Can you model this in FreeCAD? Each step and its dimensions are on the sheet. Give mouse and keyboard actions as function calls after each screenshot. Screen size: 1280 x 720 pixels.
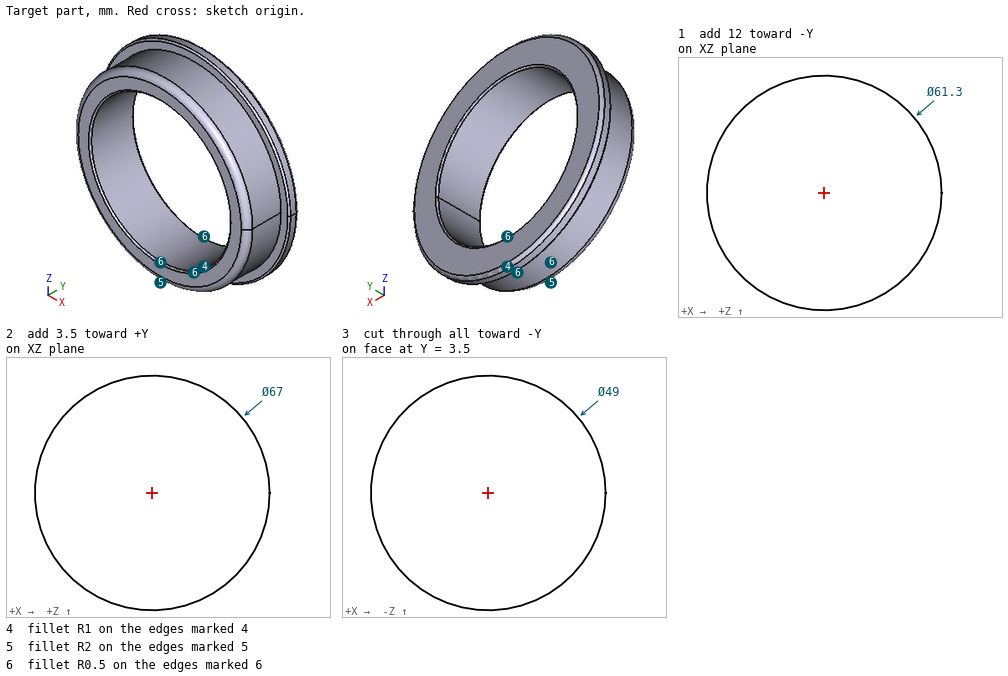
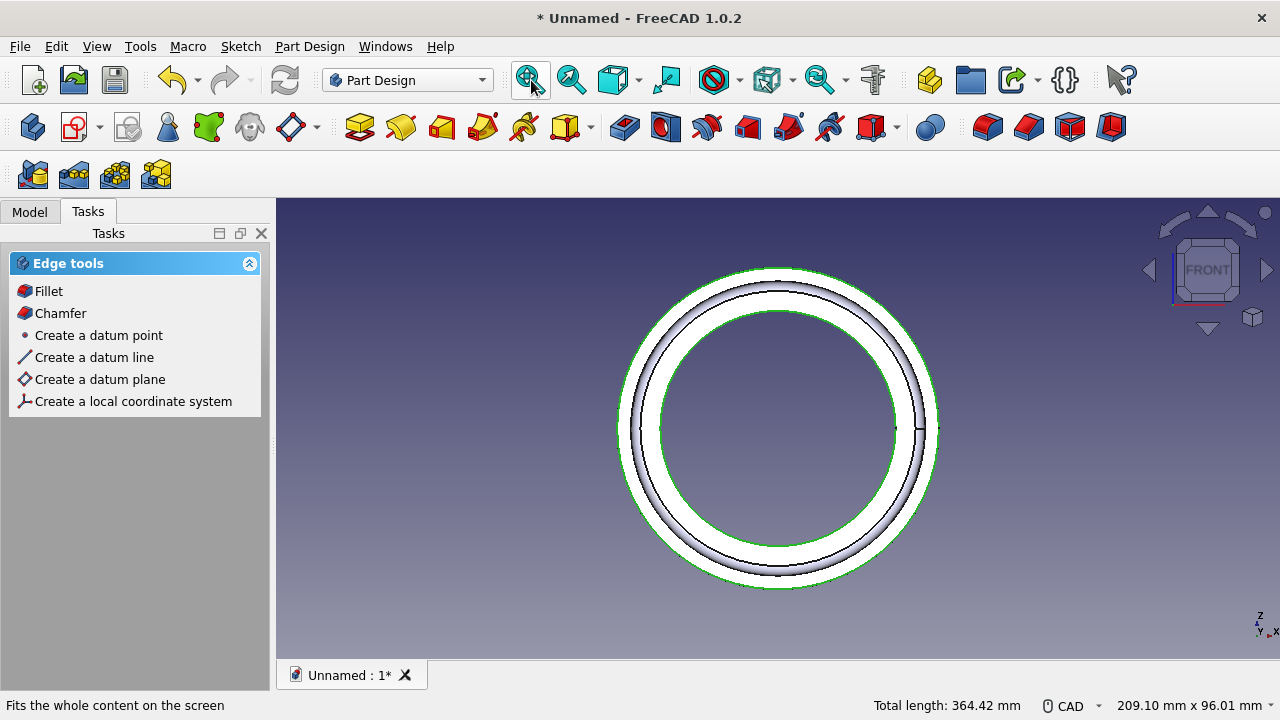
key(3)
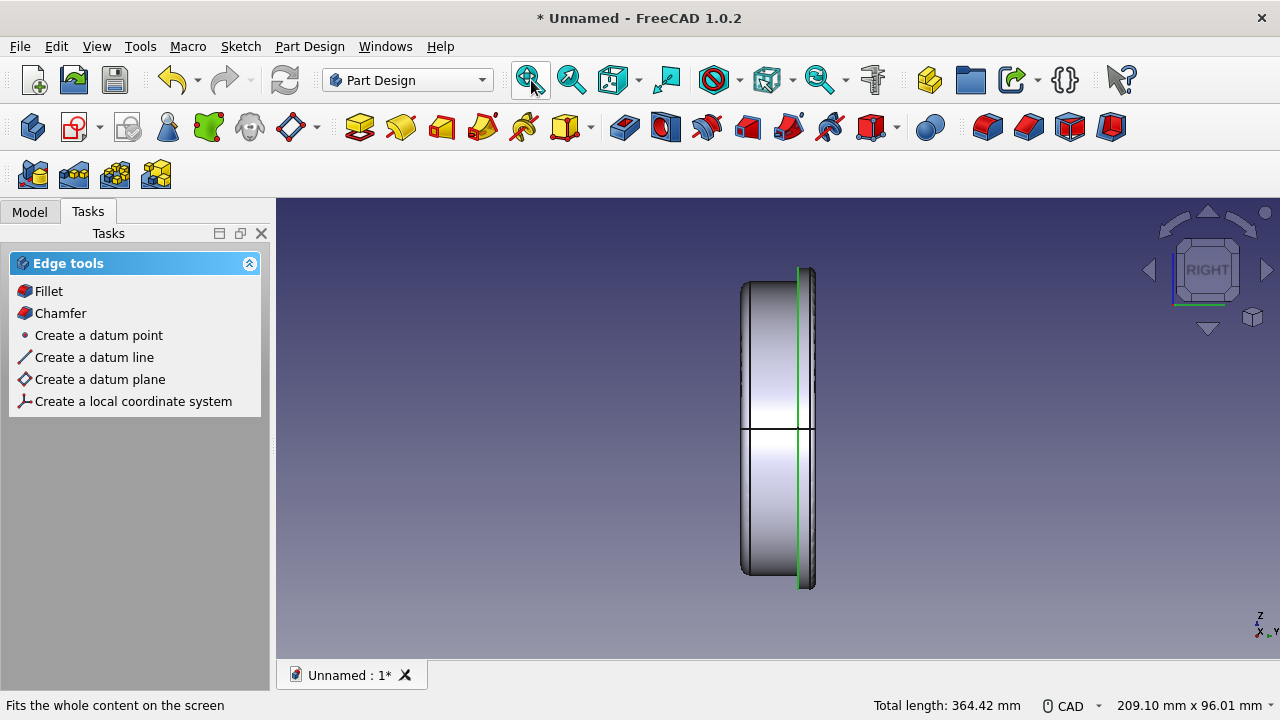
key(5)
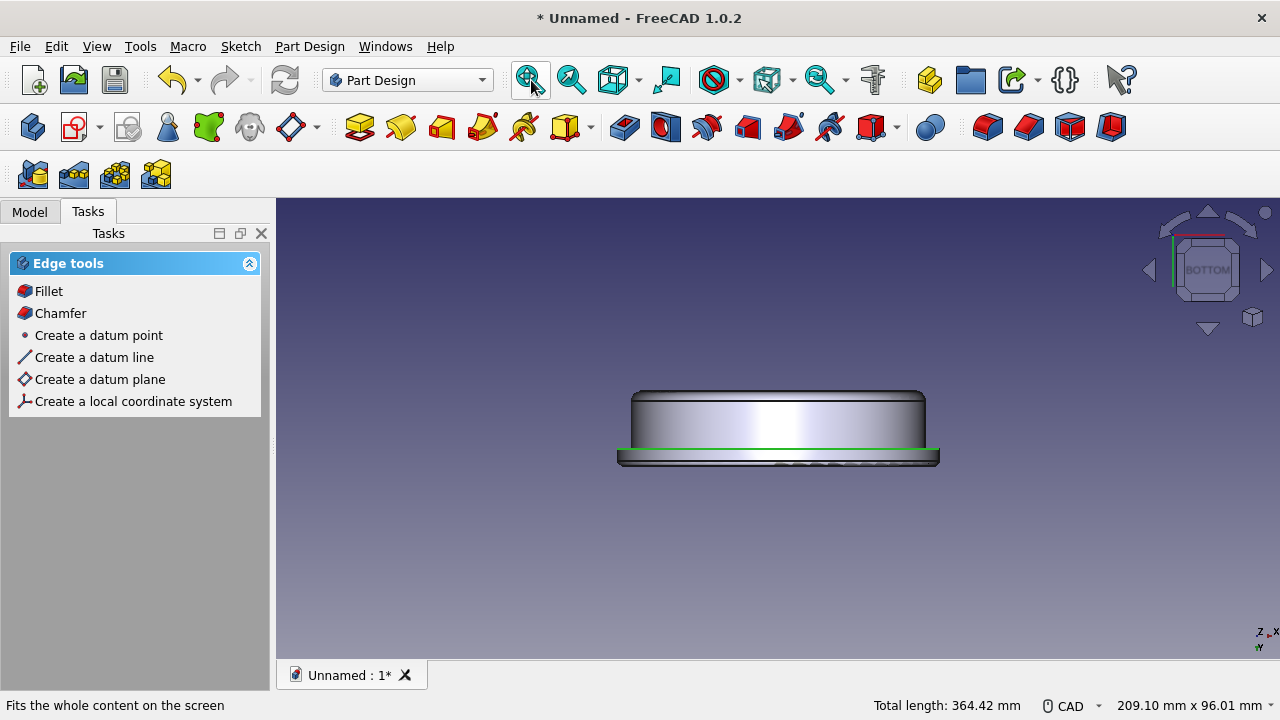
click(531, 80)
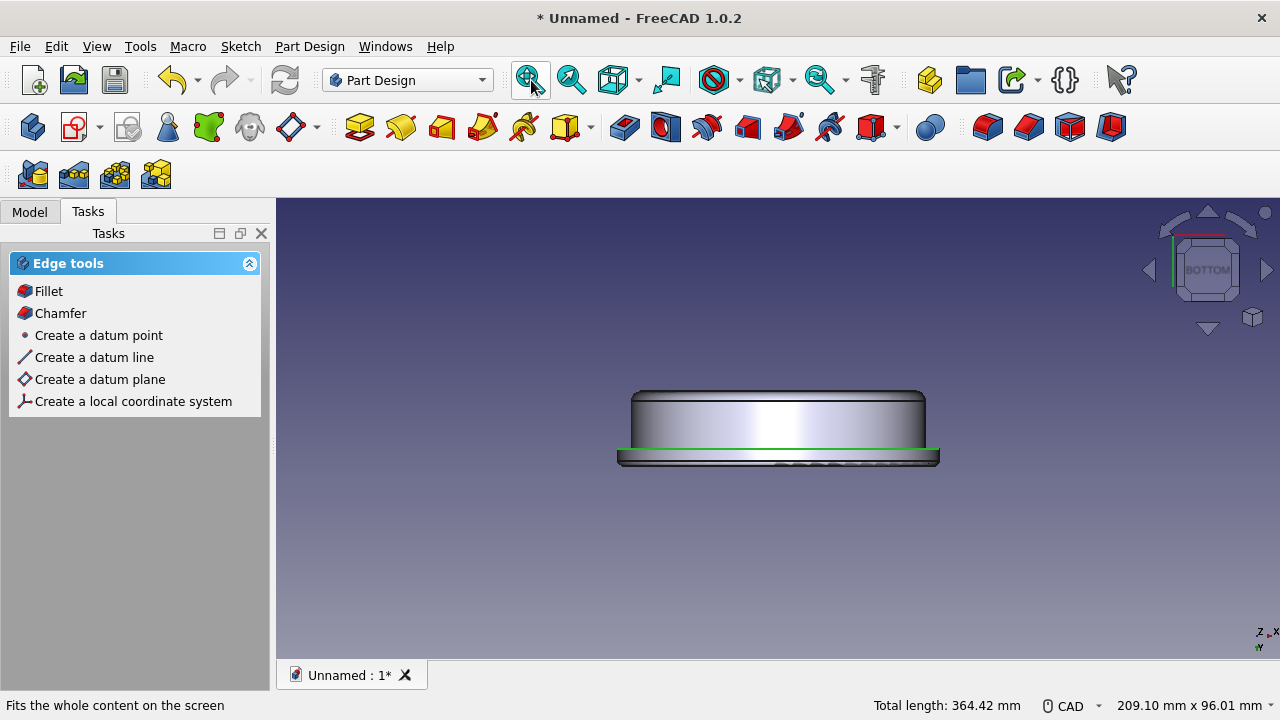
key(4)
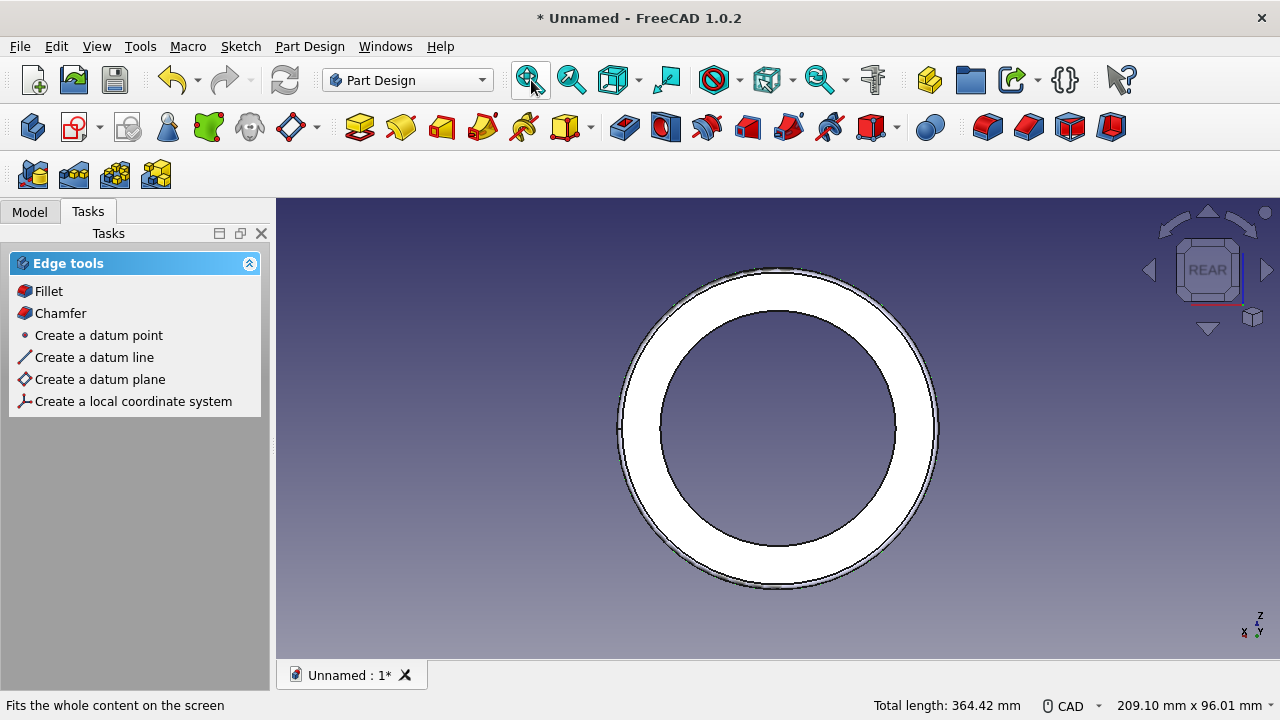
click(873, 358, ctrl)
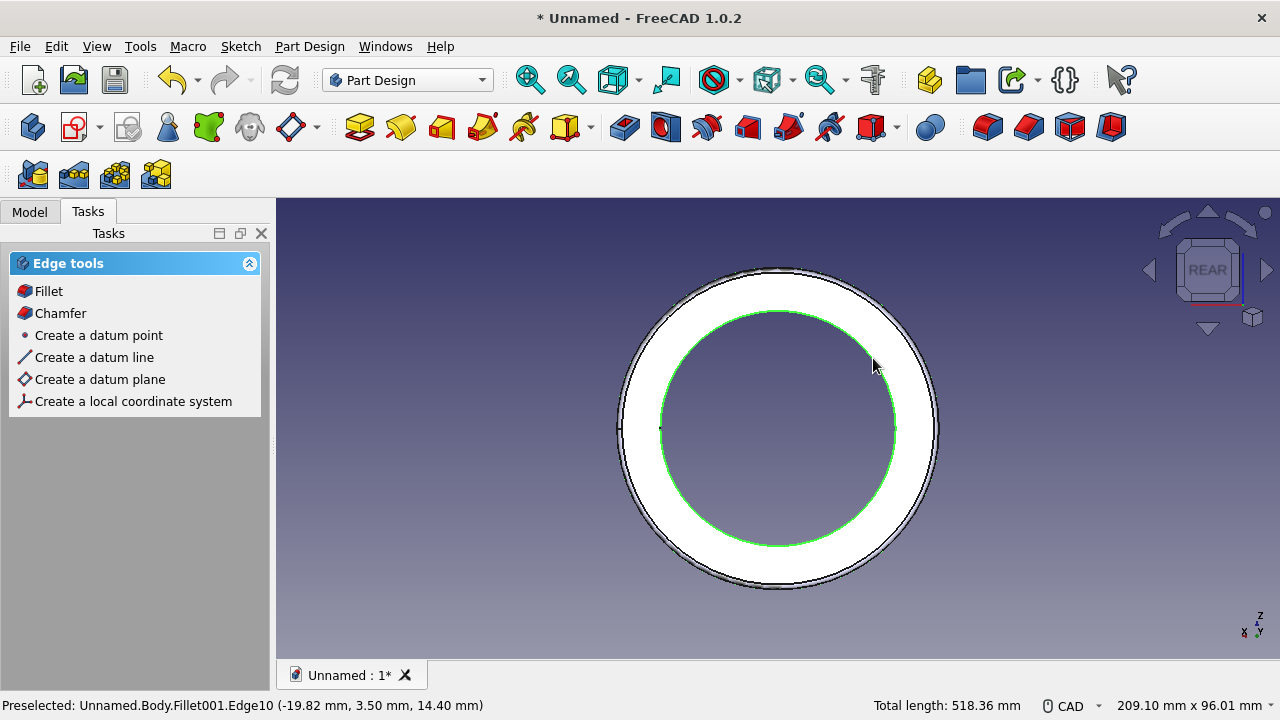
click(988, 128)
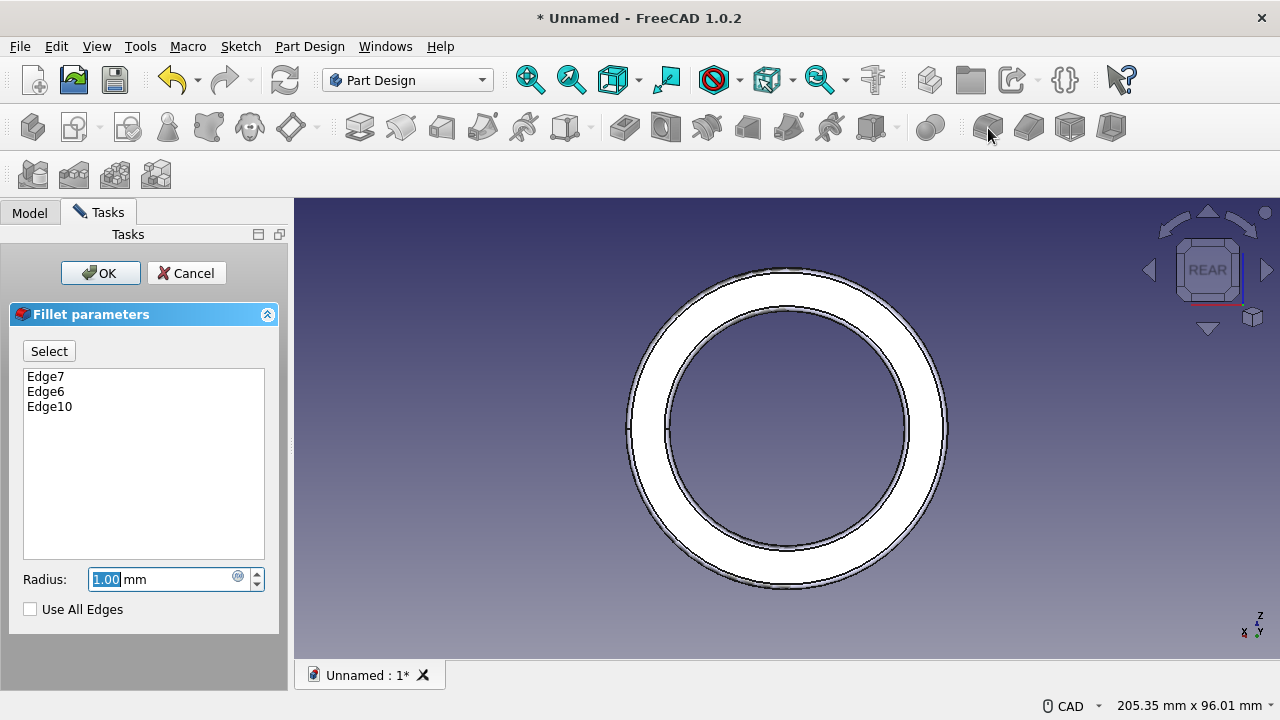
text(0.5)
key(Tab)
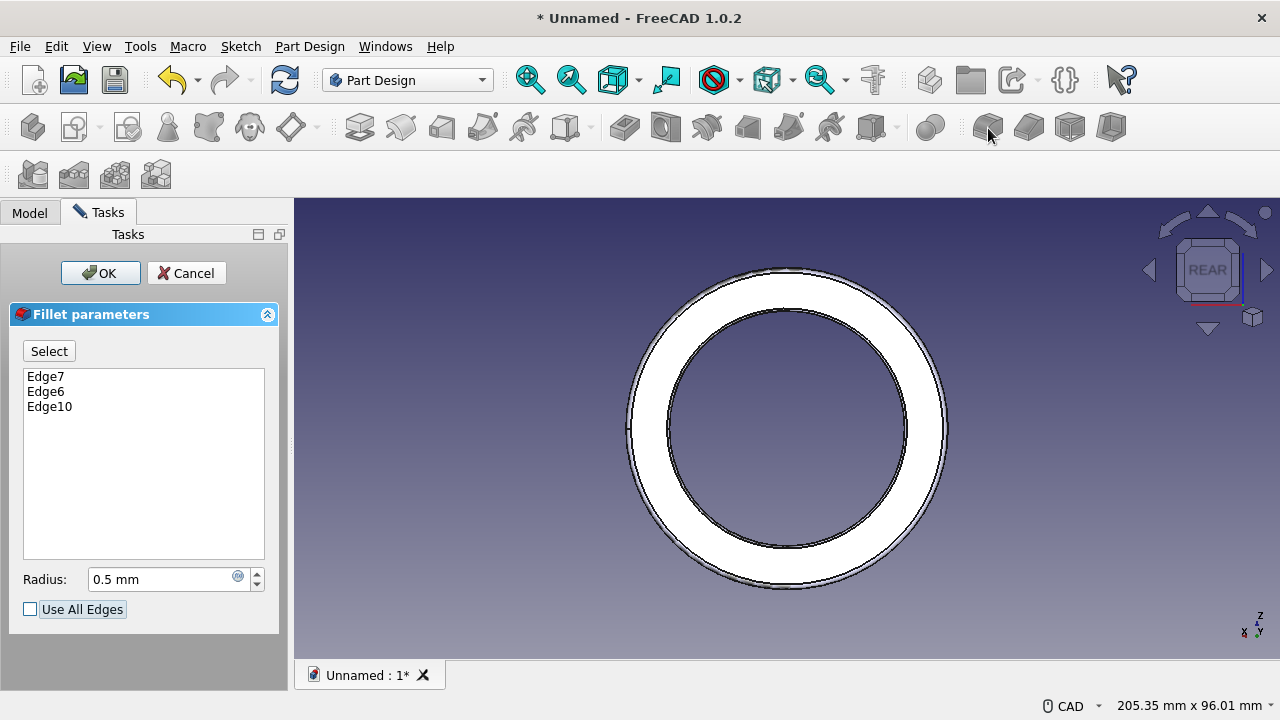
click(101, 273)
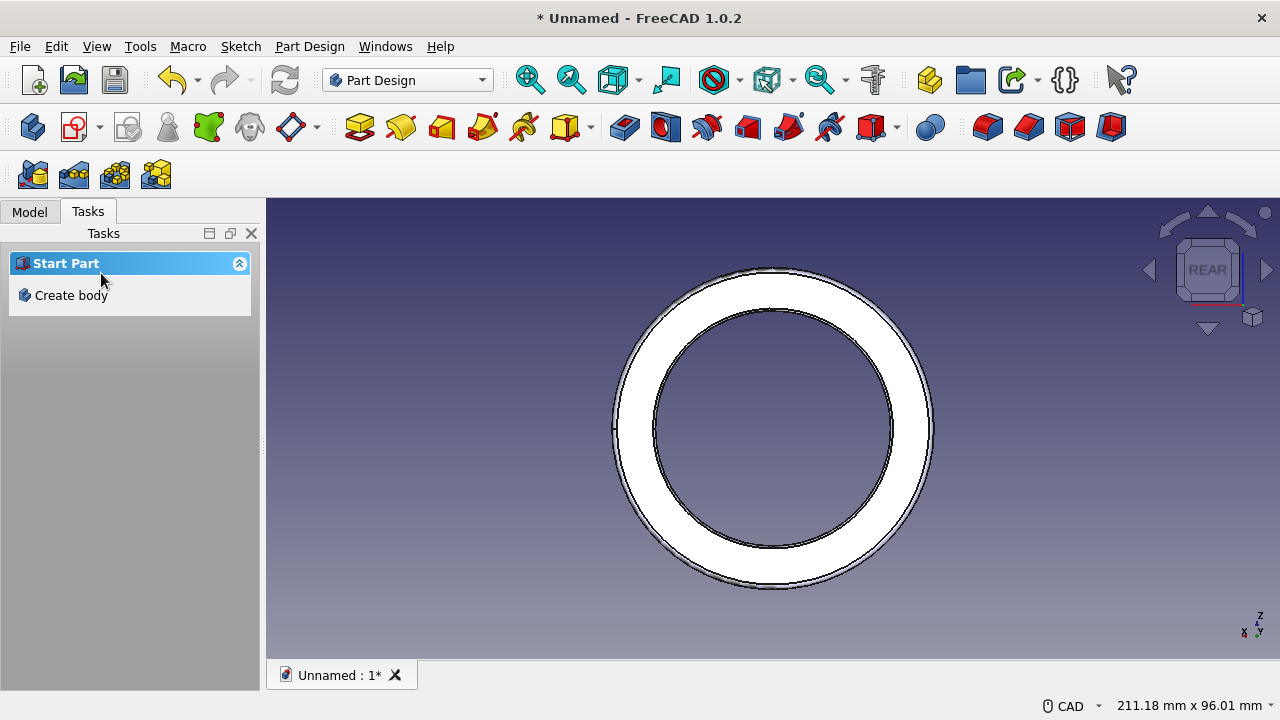
key(0)